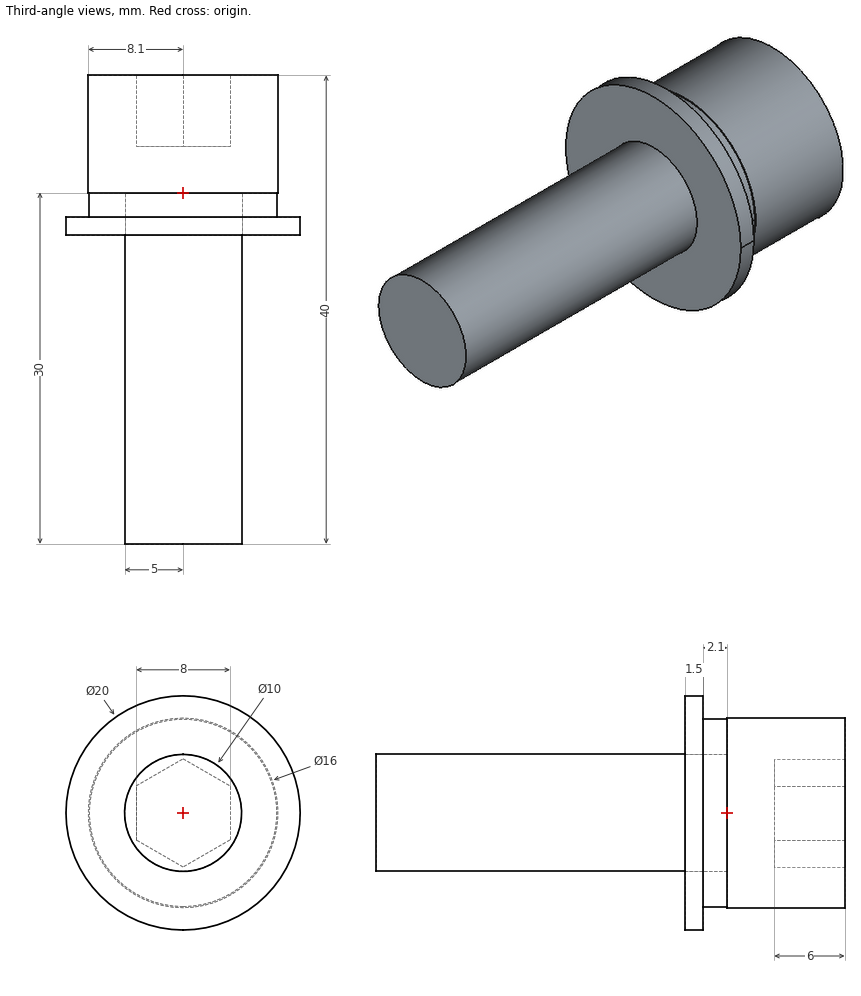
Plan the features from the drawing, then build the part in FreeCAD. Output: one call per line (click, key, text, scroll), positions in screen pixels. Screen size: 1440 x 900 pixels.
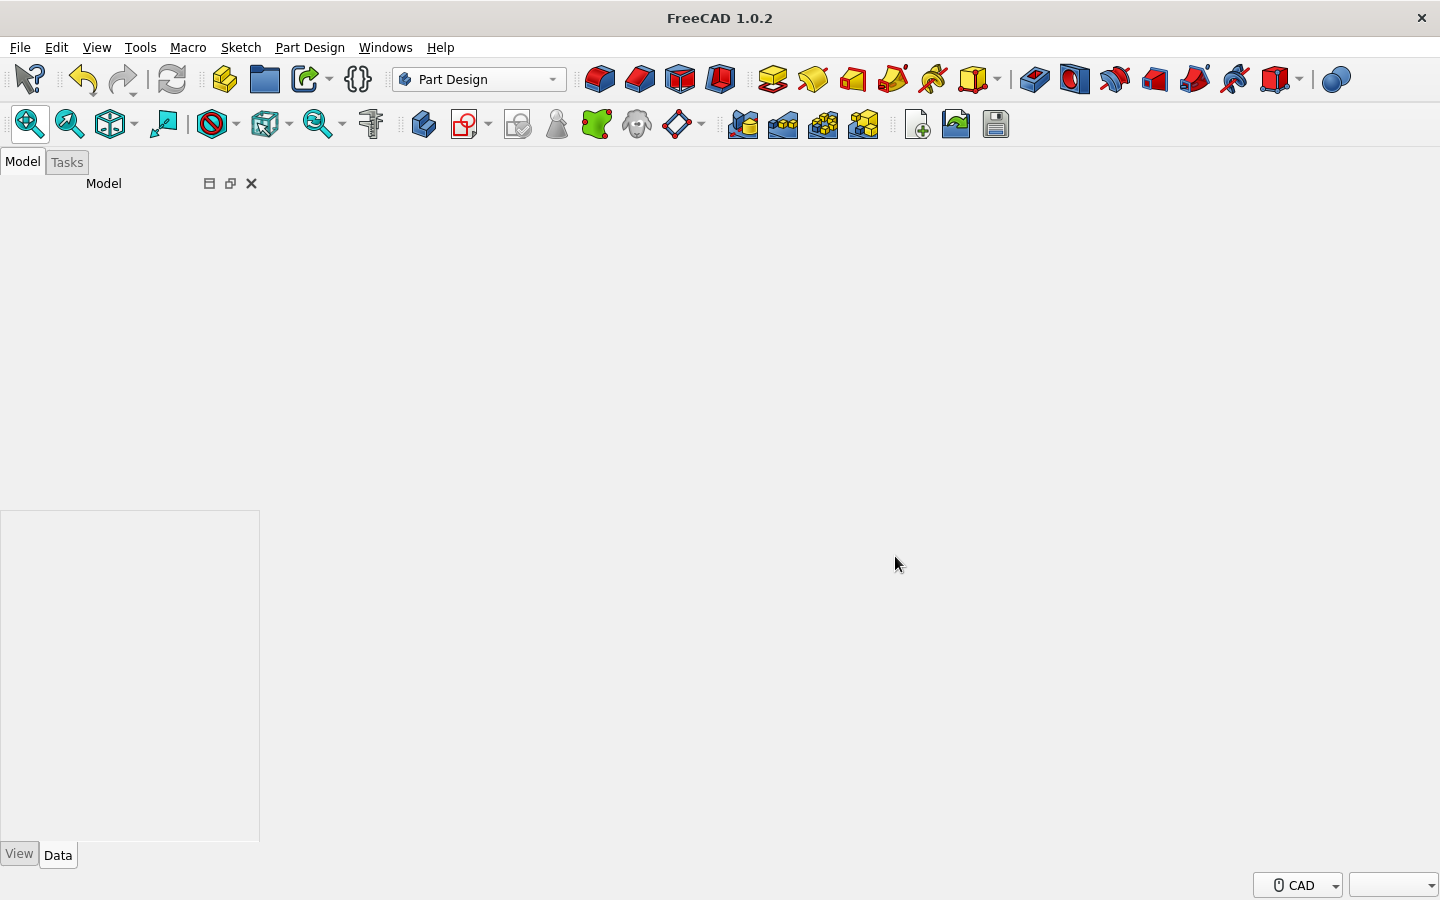
click(916, 124)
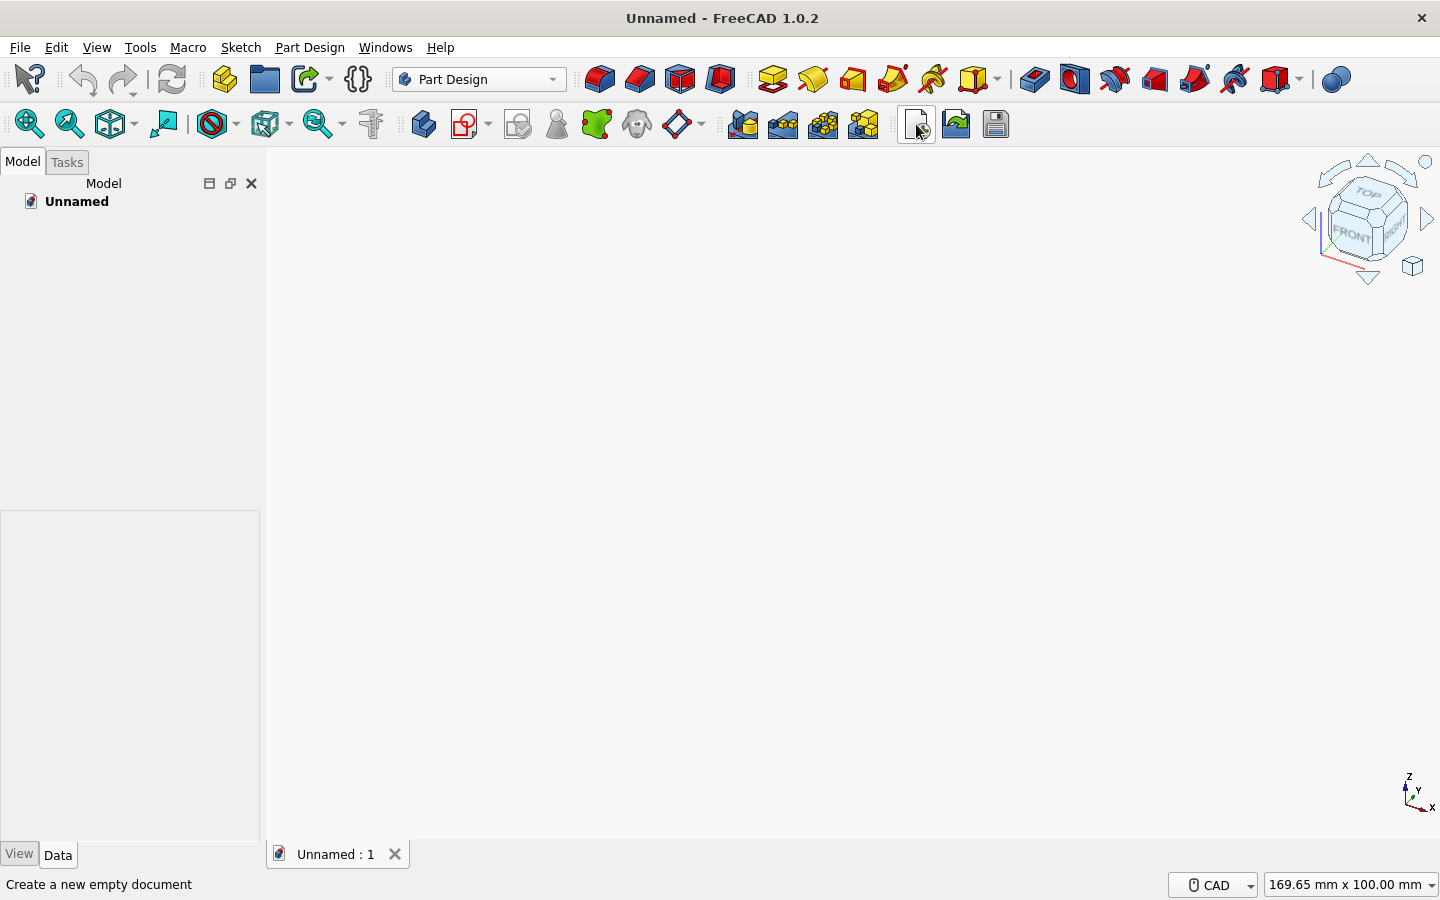
click(464, 124)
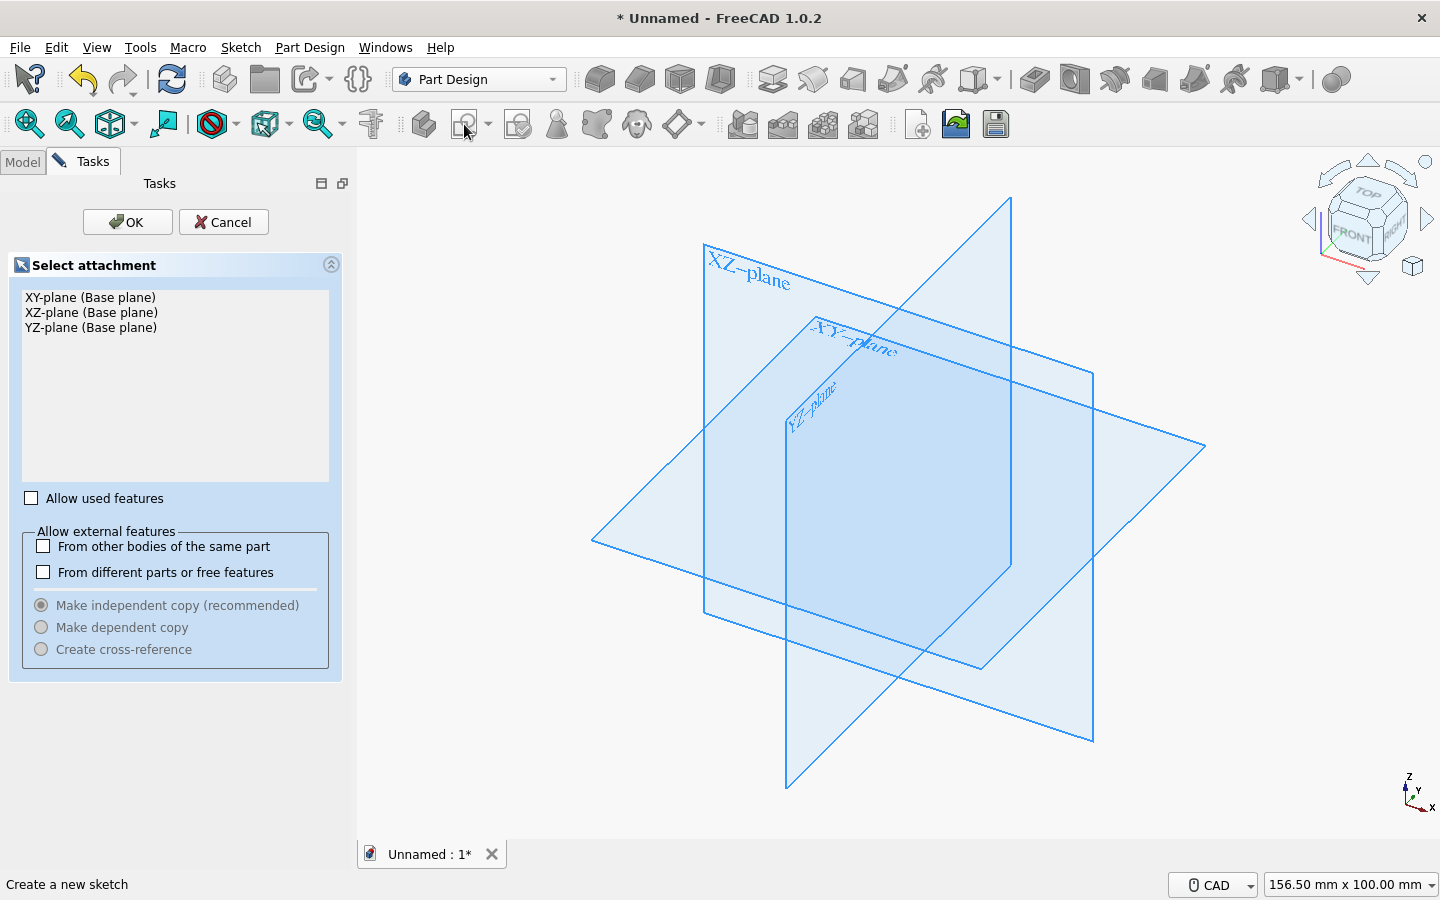
click(82, 298)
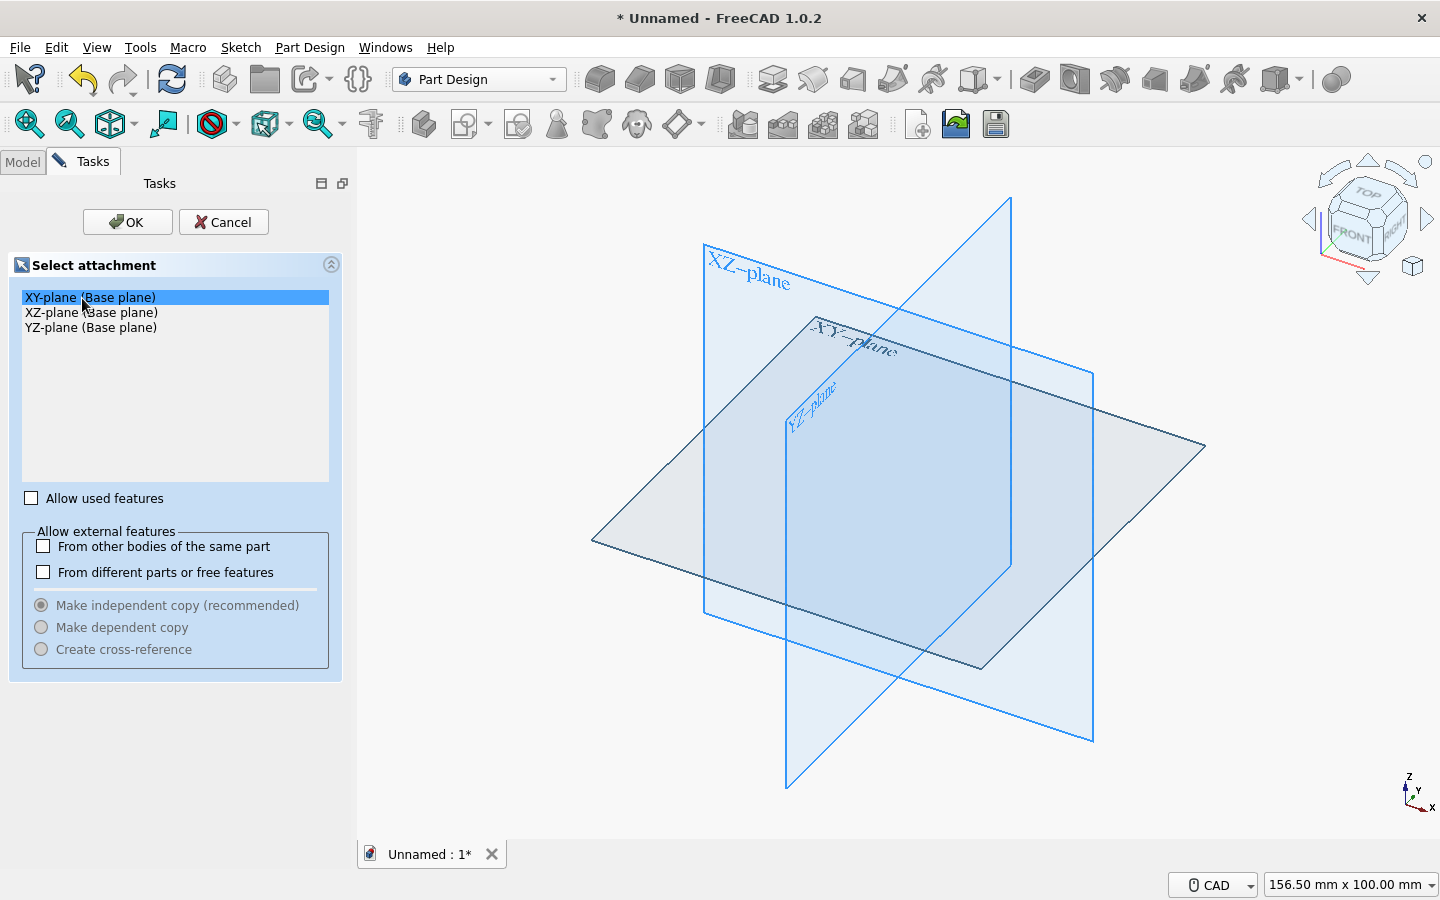
click(128, 222)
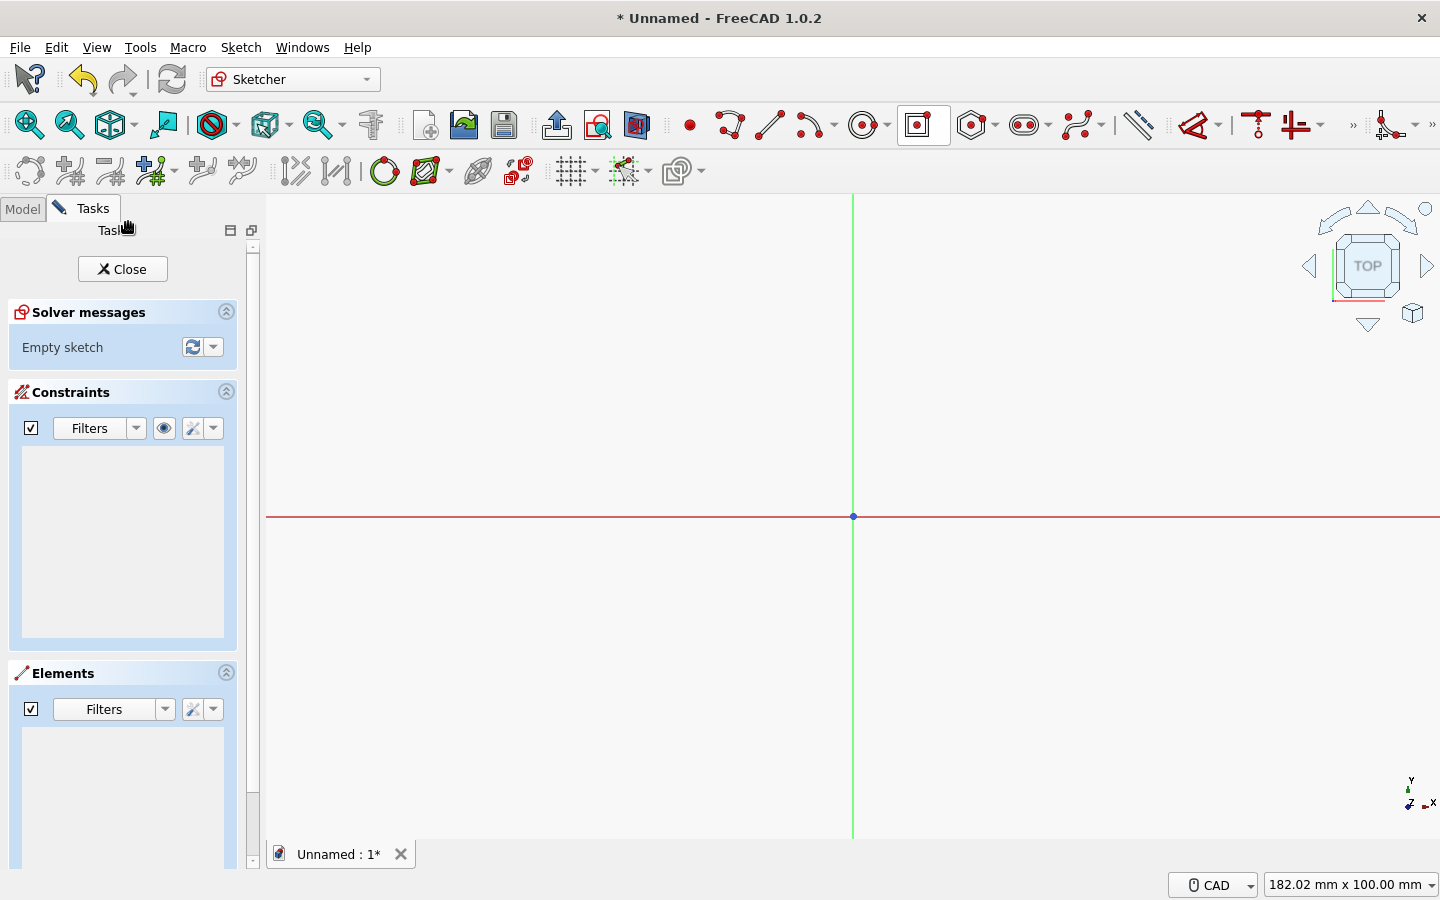
scroll(913, 712, up, 2)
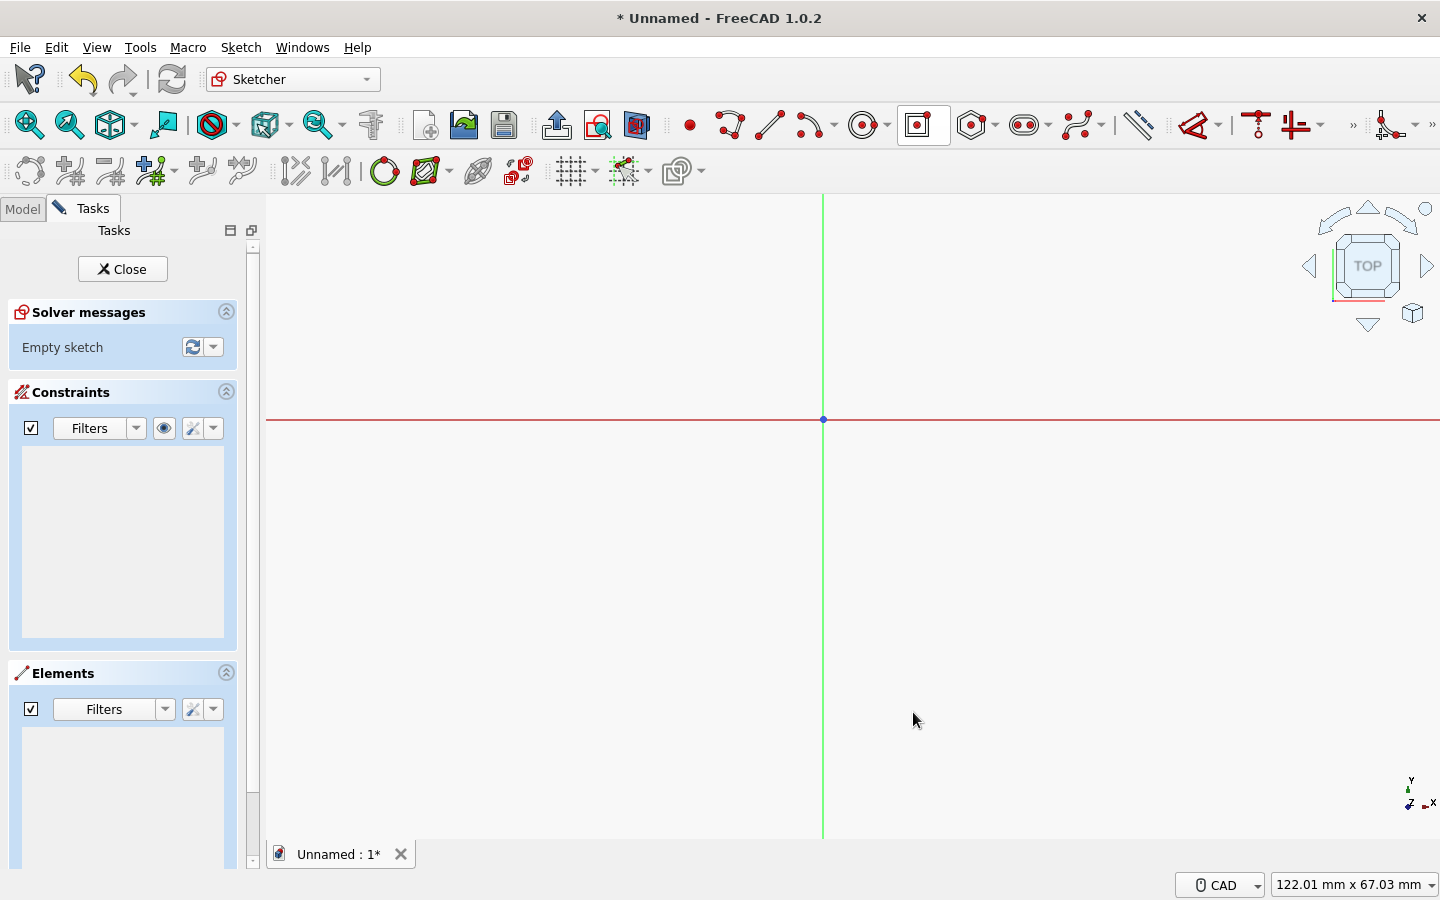
key(g)
key(m)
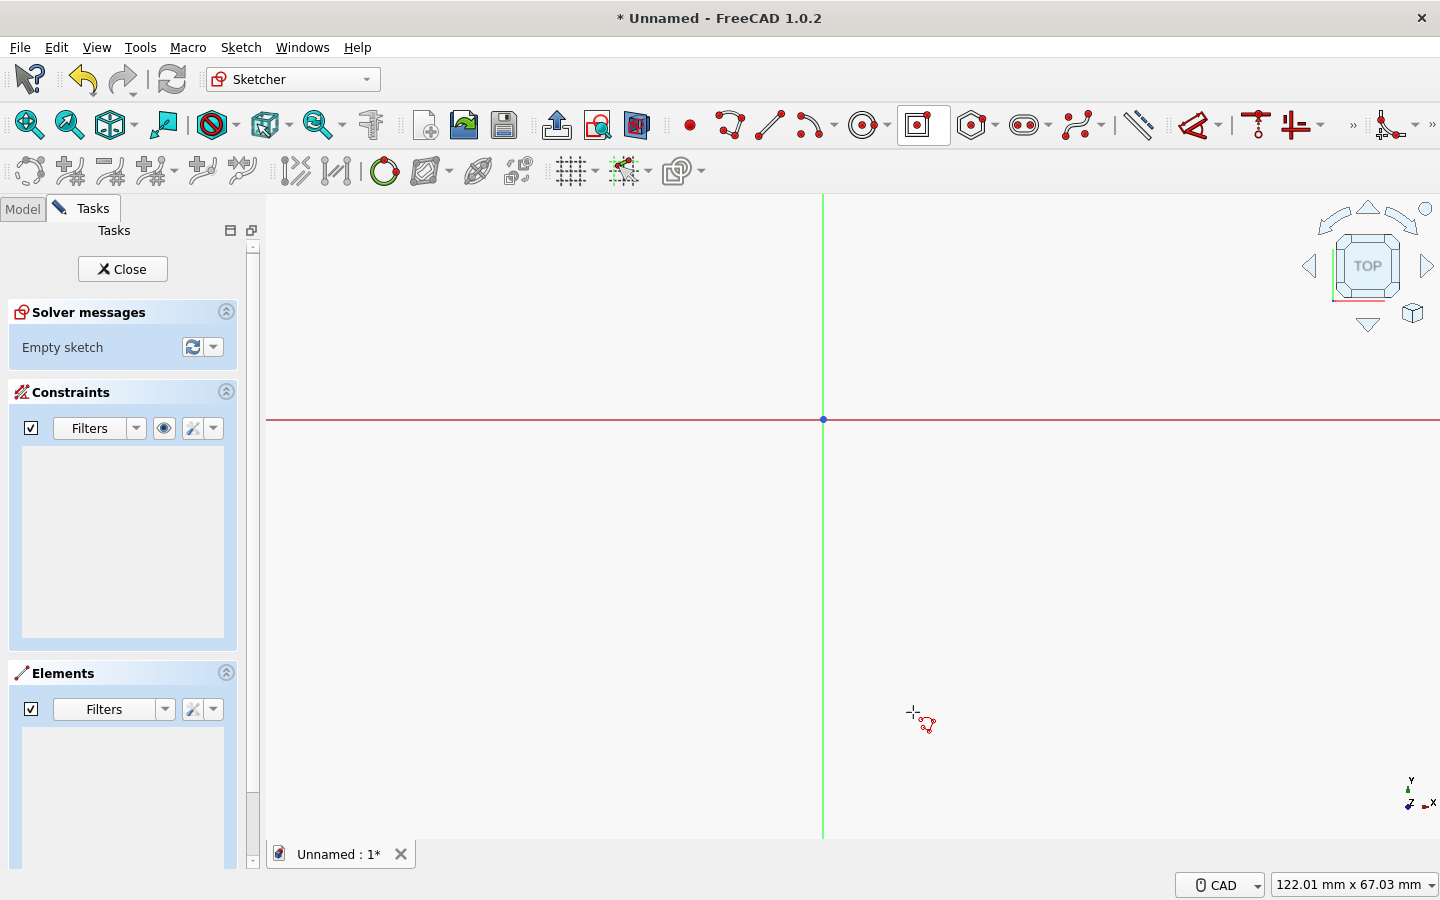
click(775, 420)
click(775, 709)
click(823, 709)
click(814, 324)
click(745, 324)
click(745, 429)
click(775, 420)
key(Escape)
key(Escape)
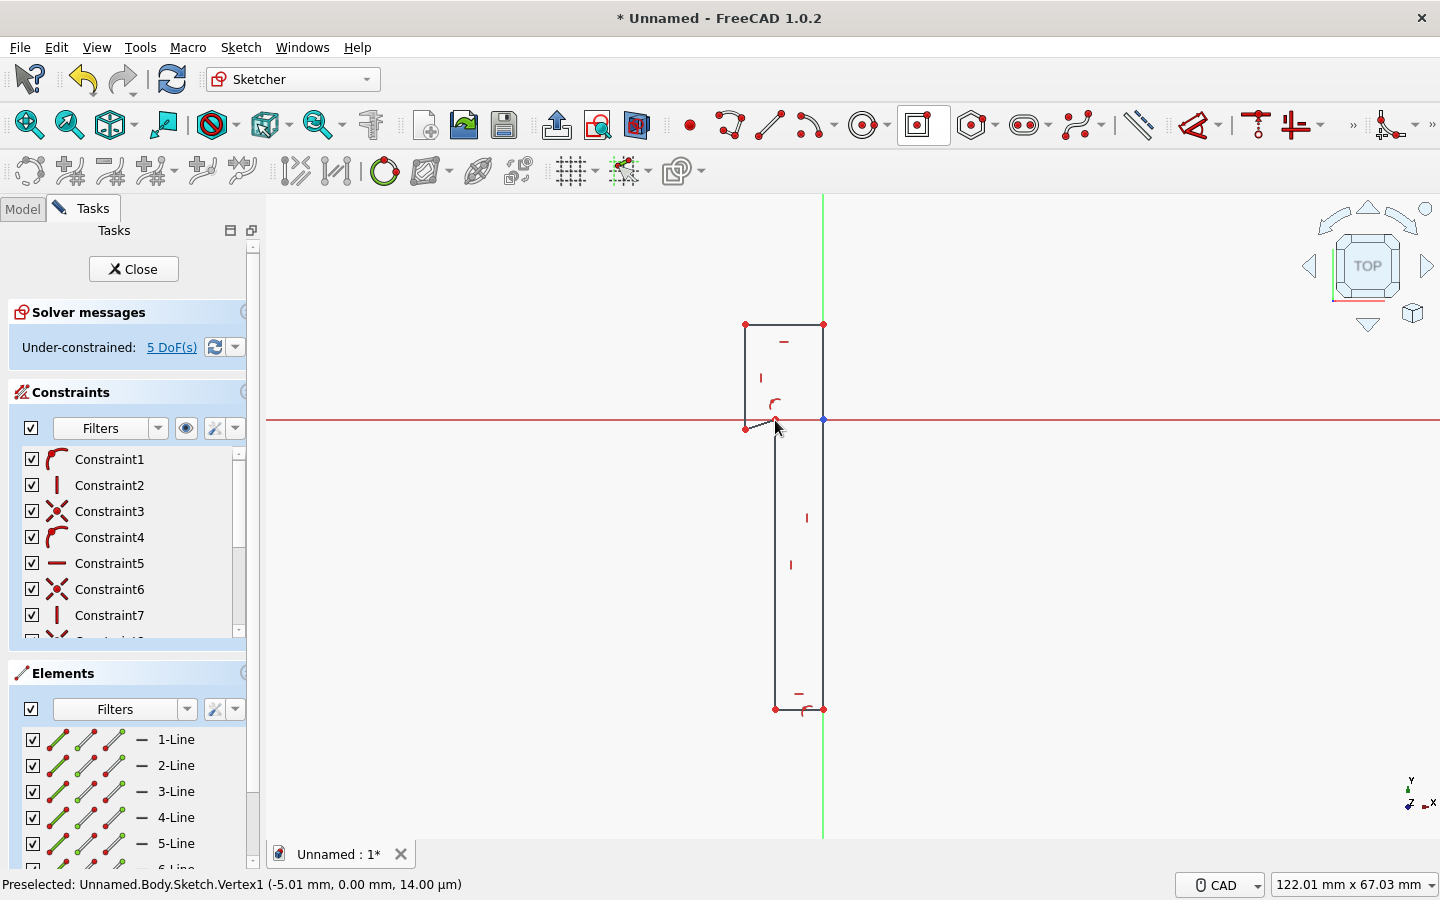
scroll(766, 423, up, 3)